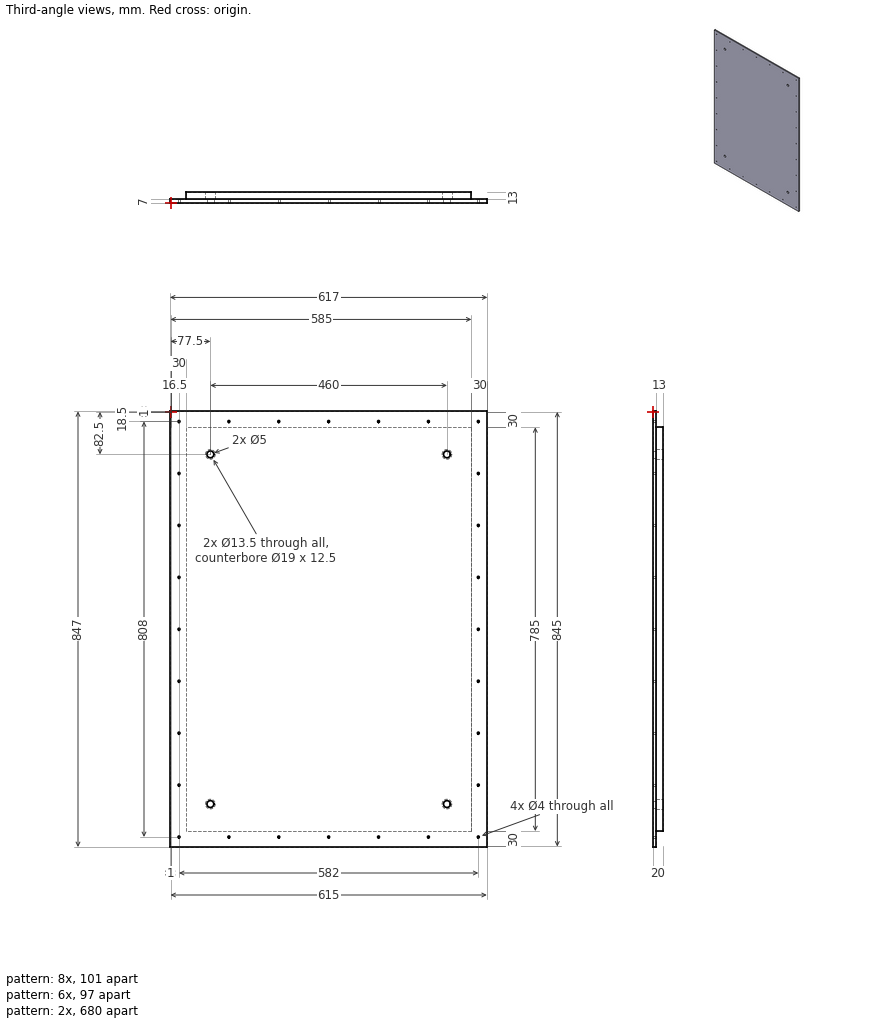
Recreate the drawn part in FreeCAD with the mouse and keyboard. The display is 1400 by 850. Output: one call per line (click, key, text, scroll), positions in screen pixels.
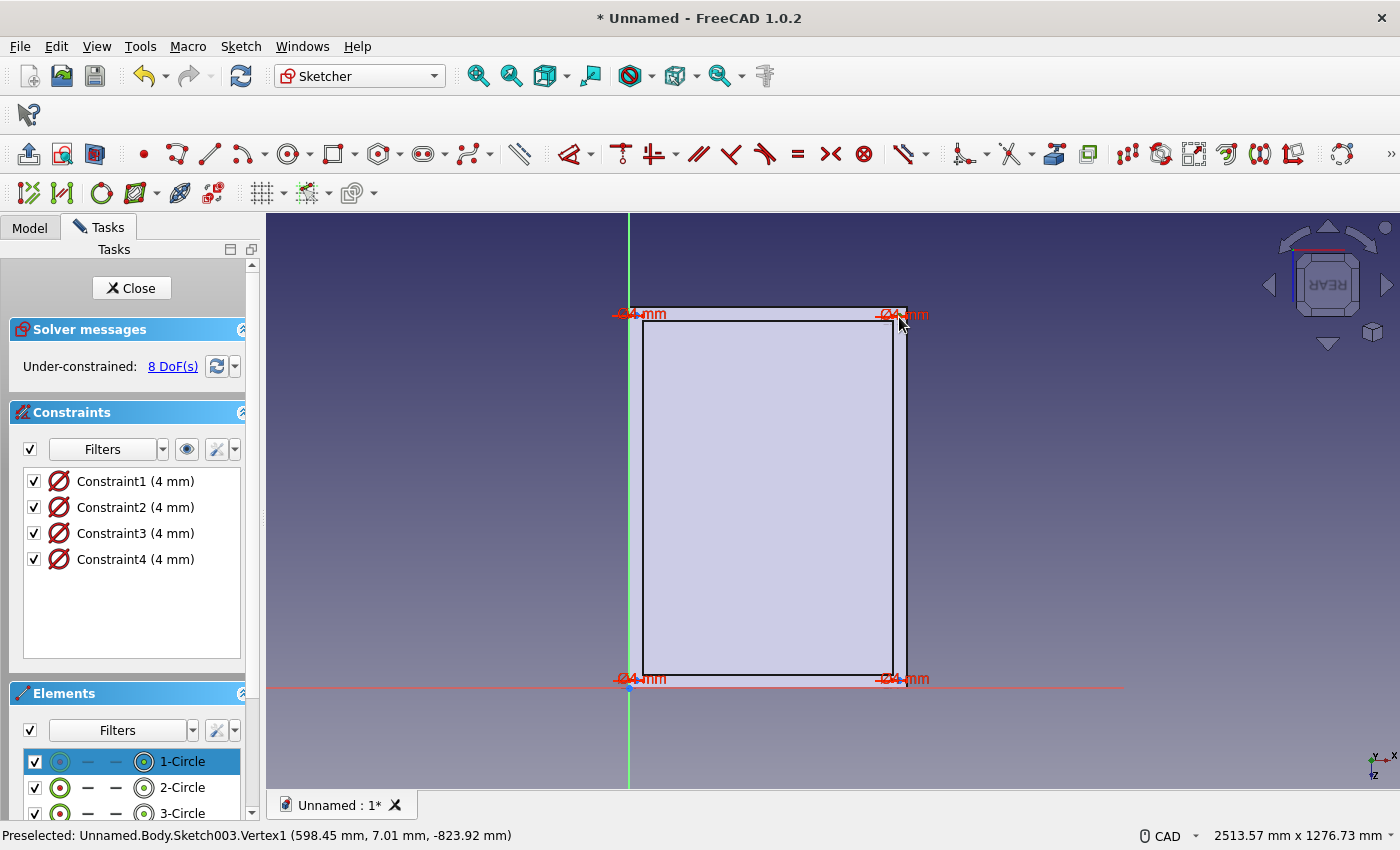
click(637, 316)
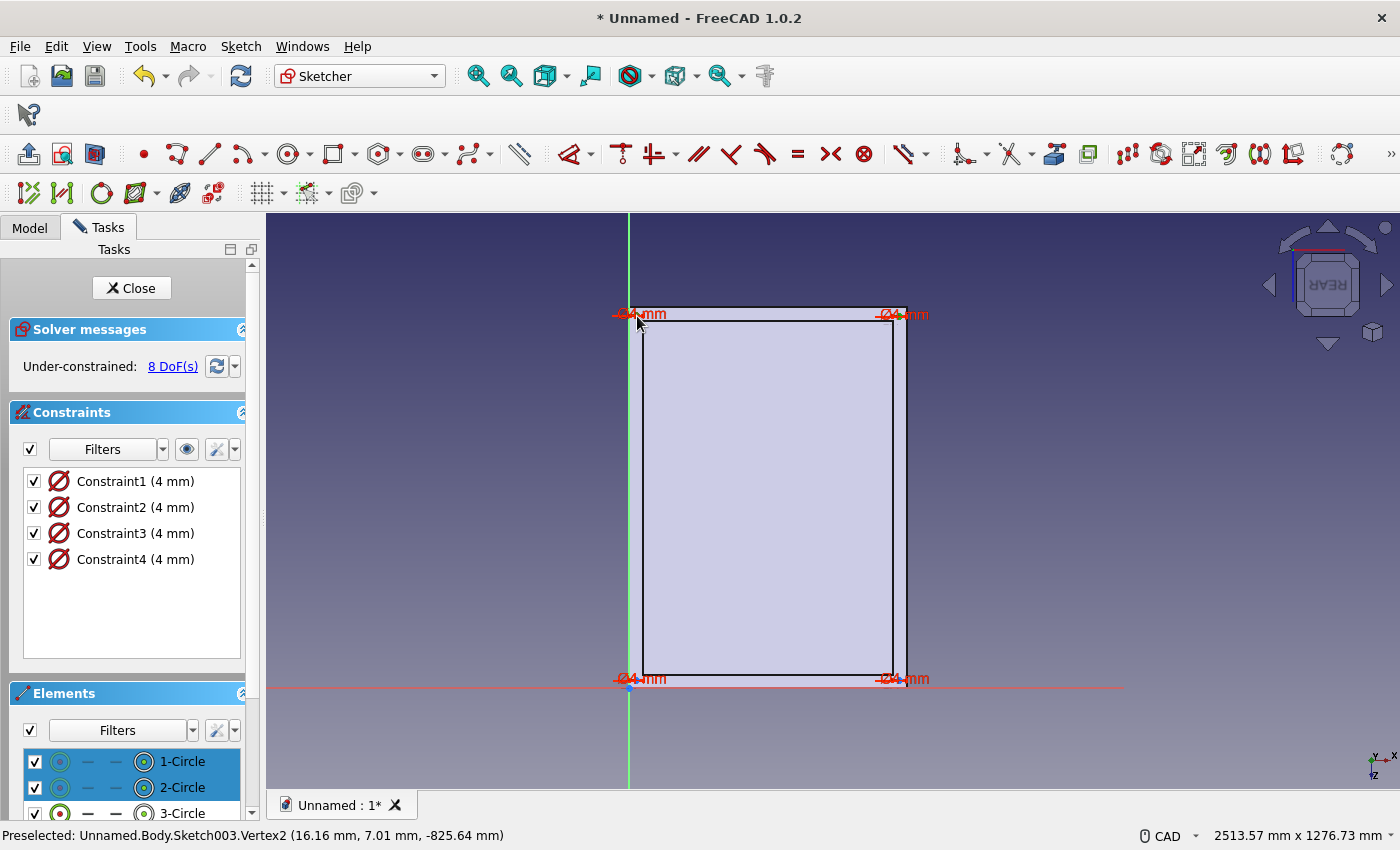
key(h)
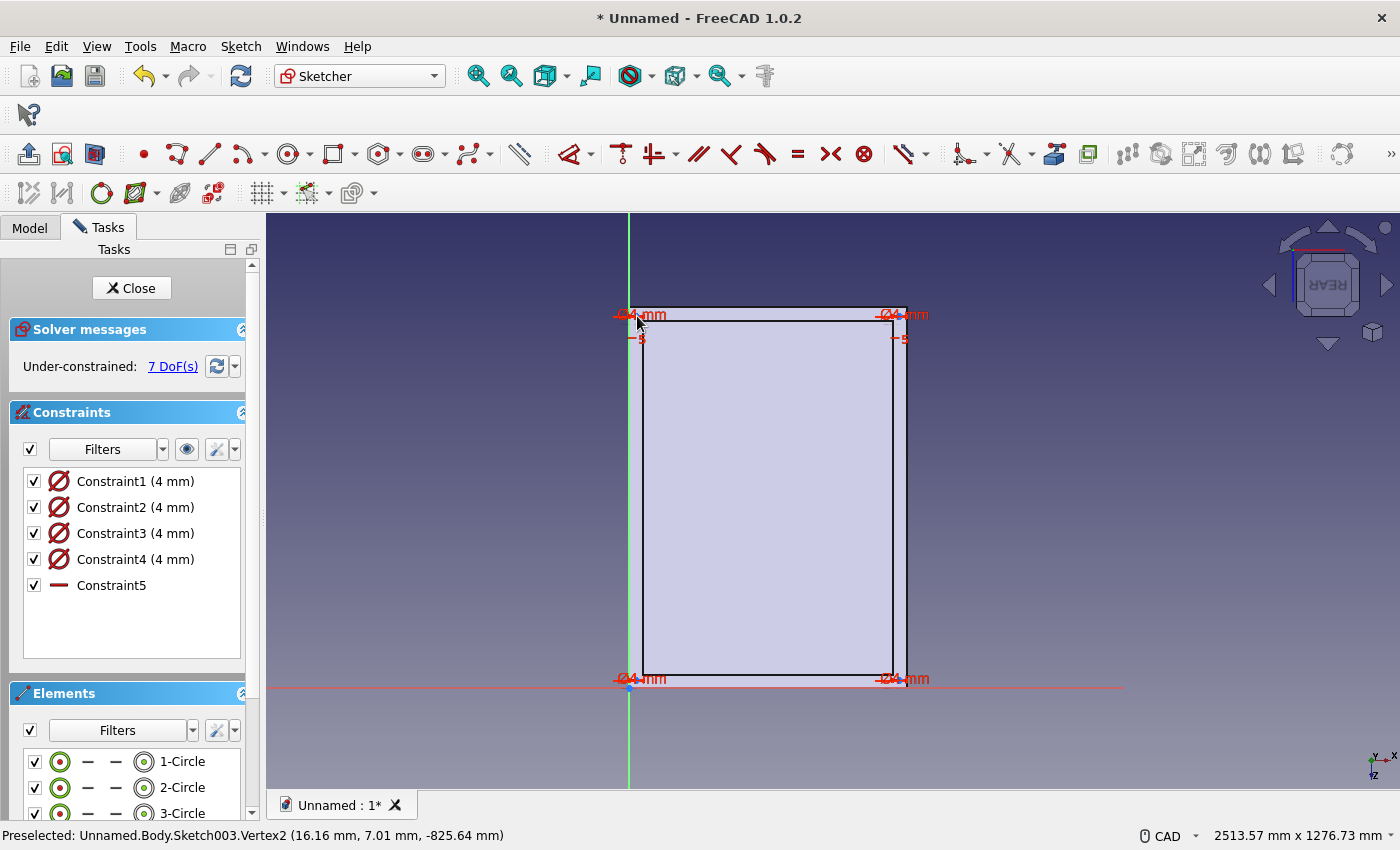
click(637, 317)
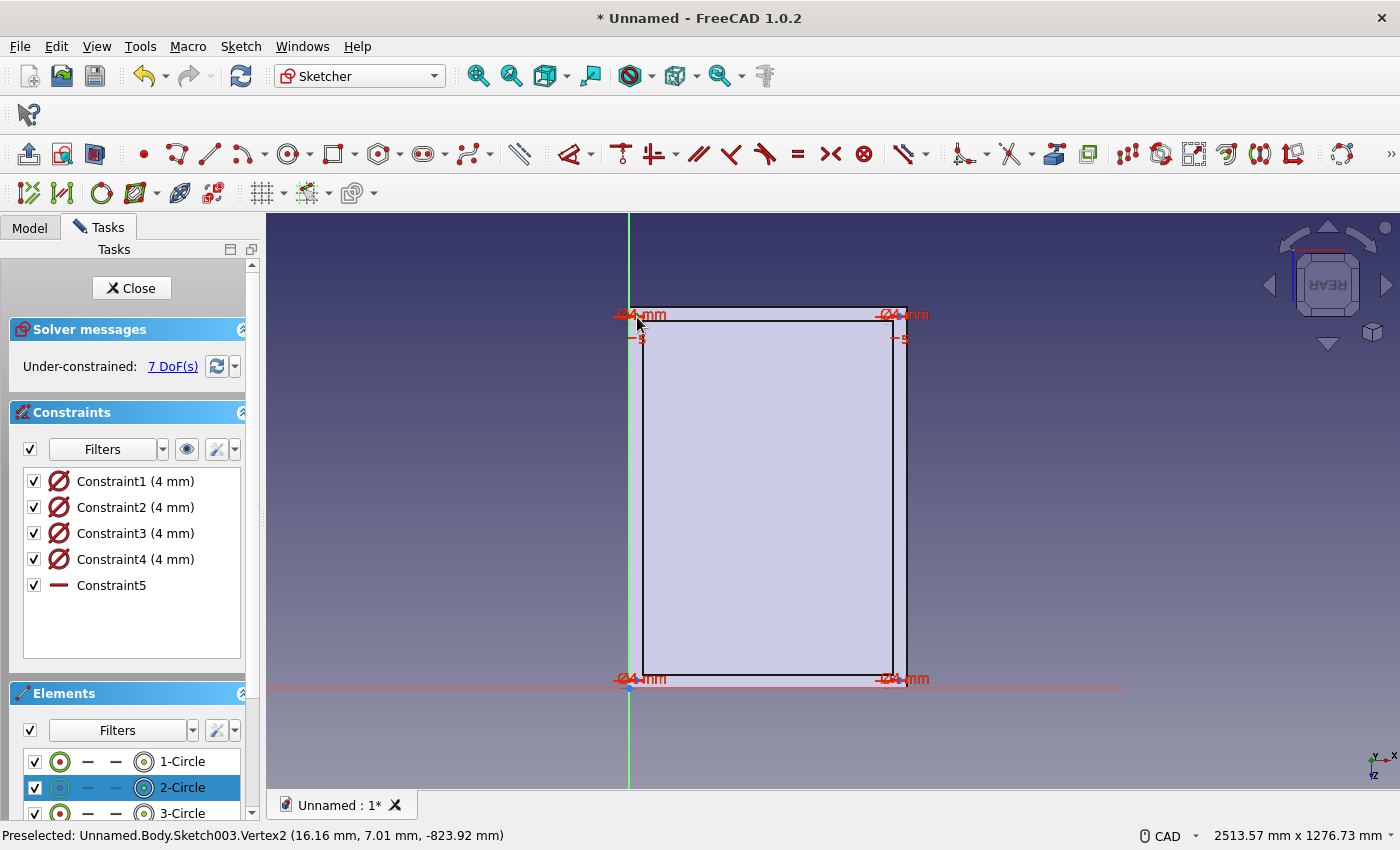
click(637, 681)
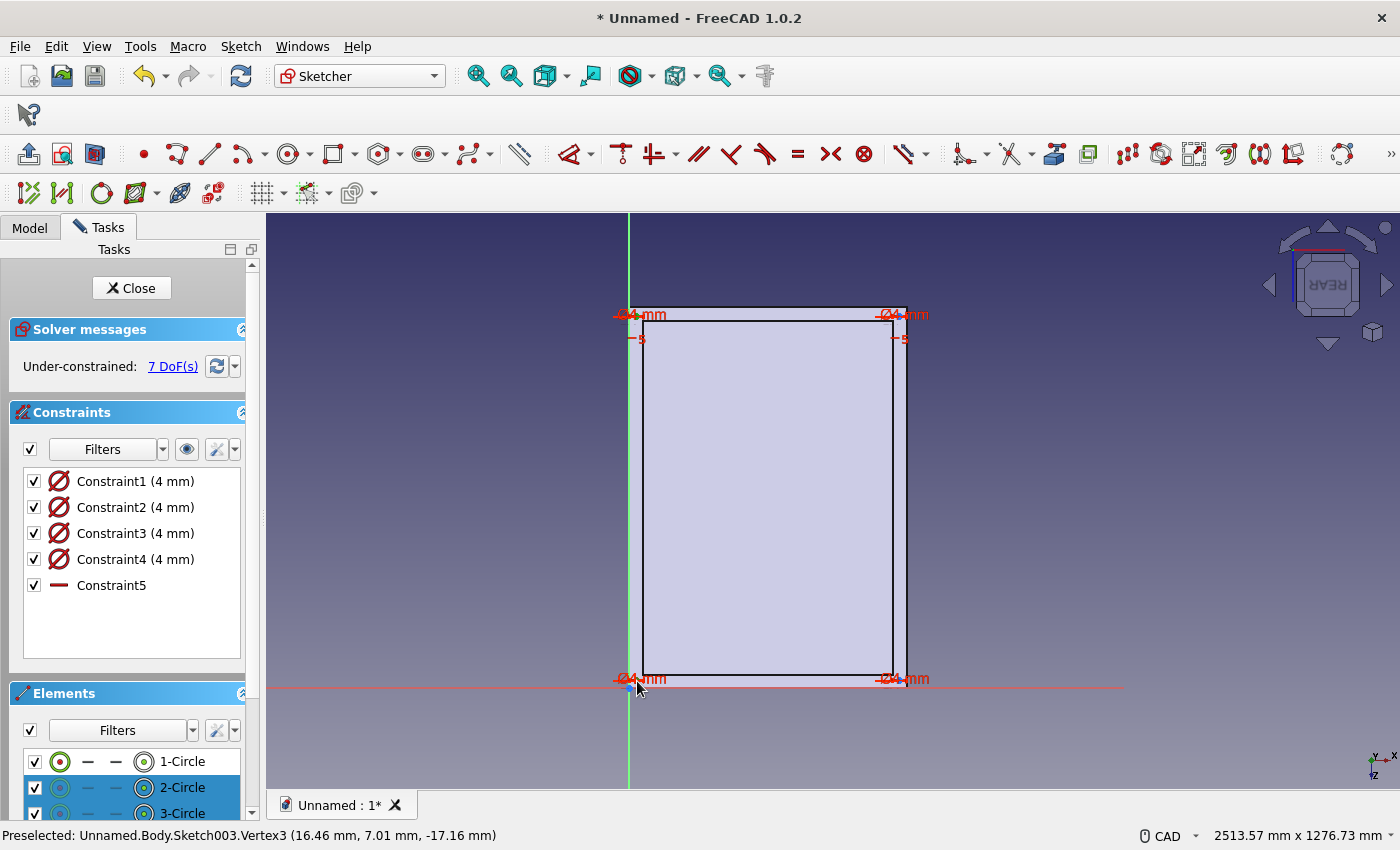
key(v)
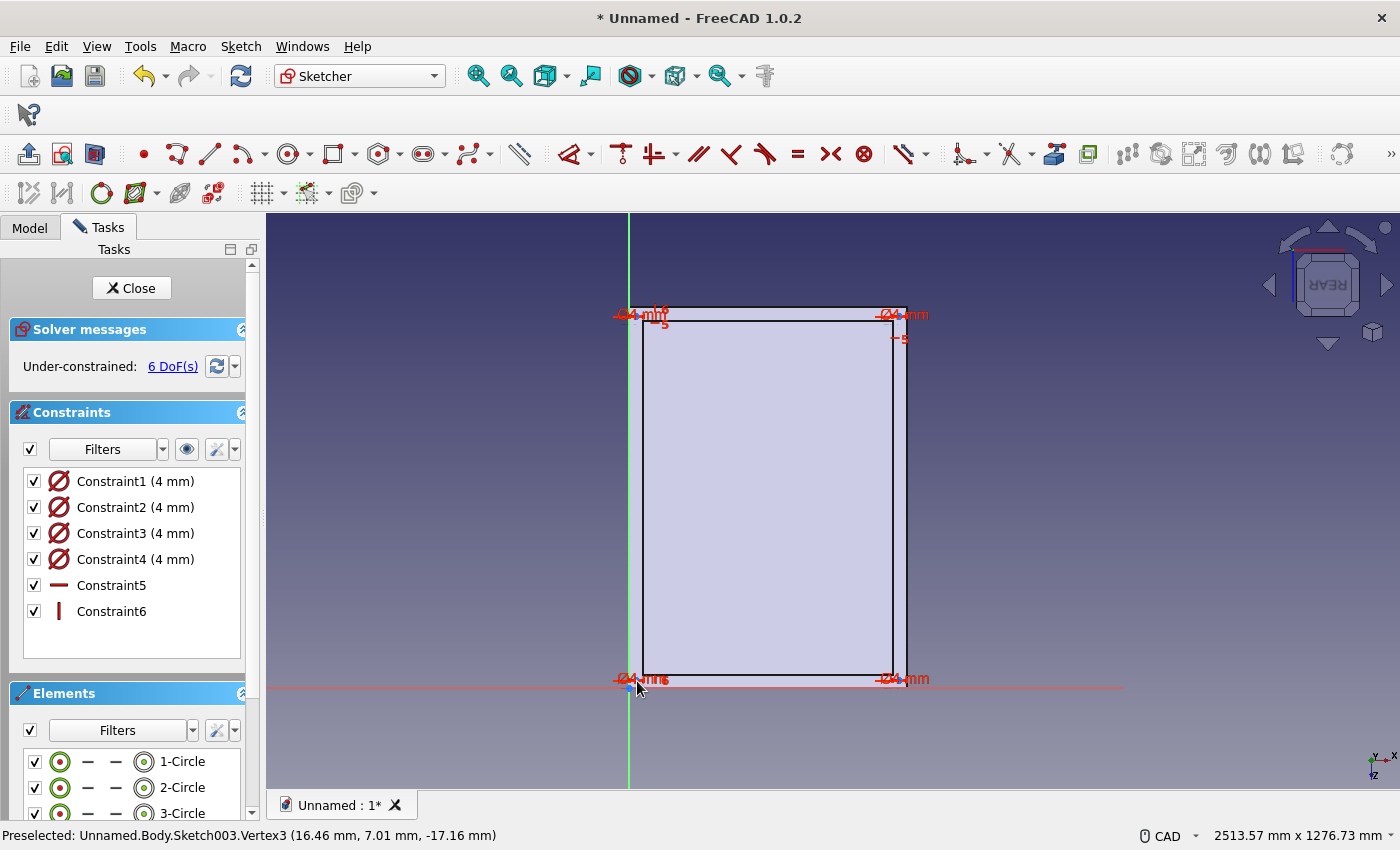
click(899, 317)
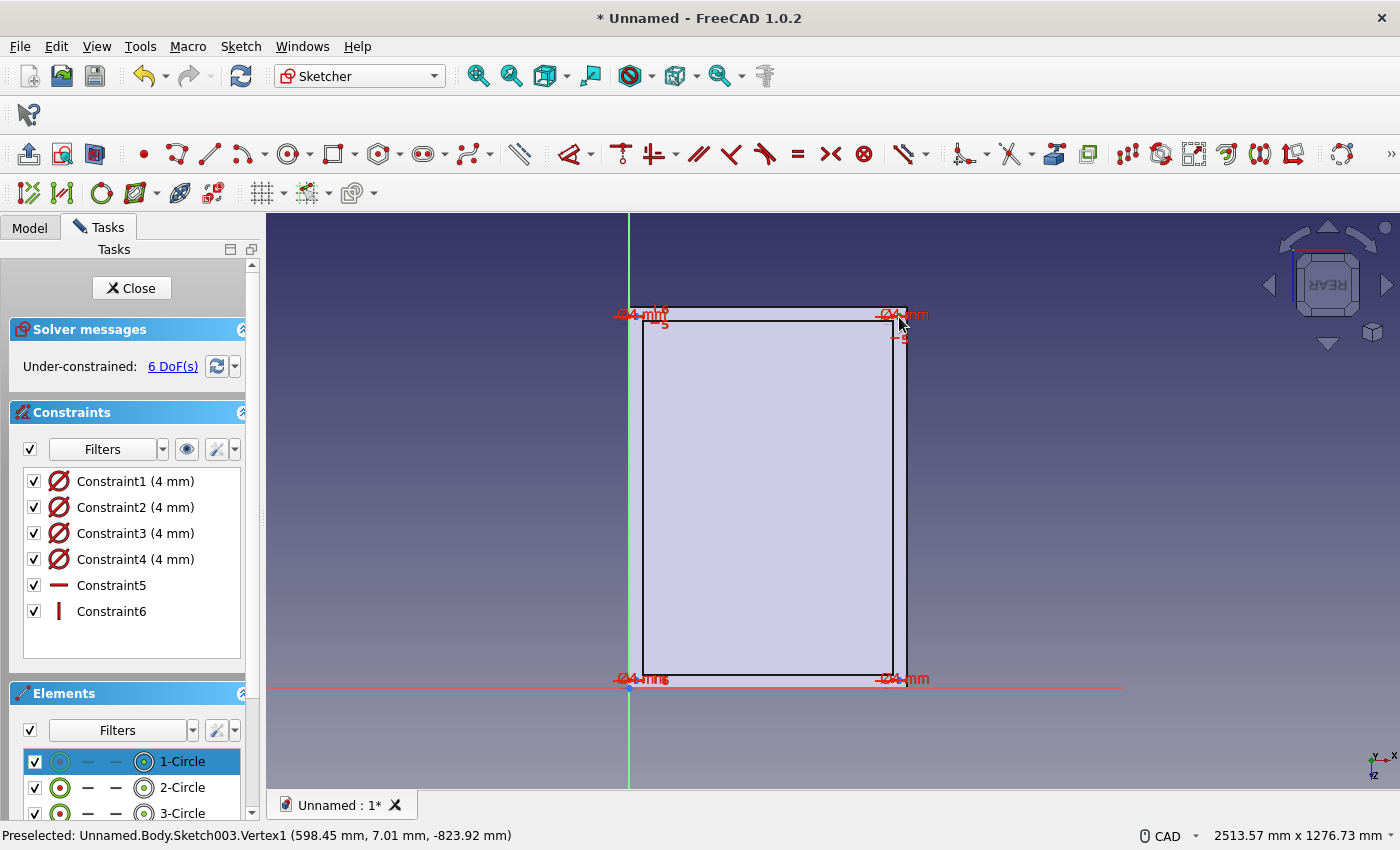
click(900, 681)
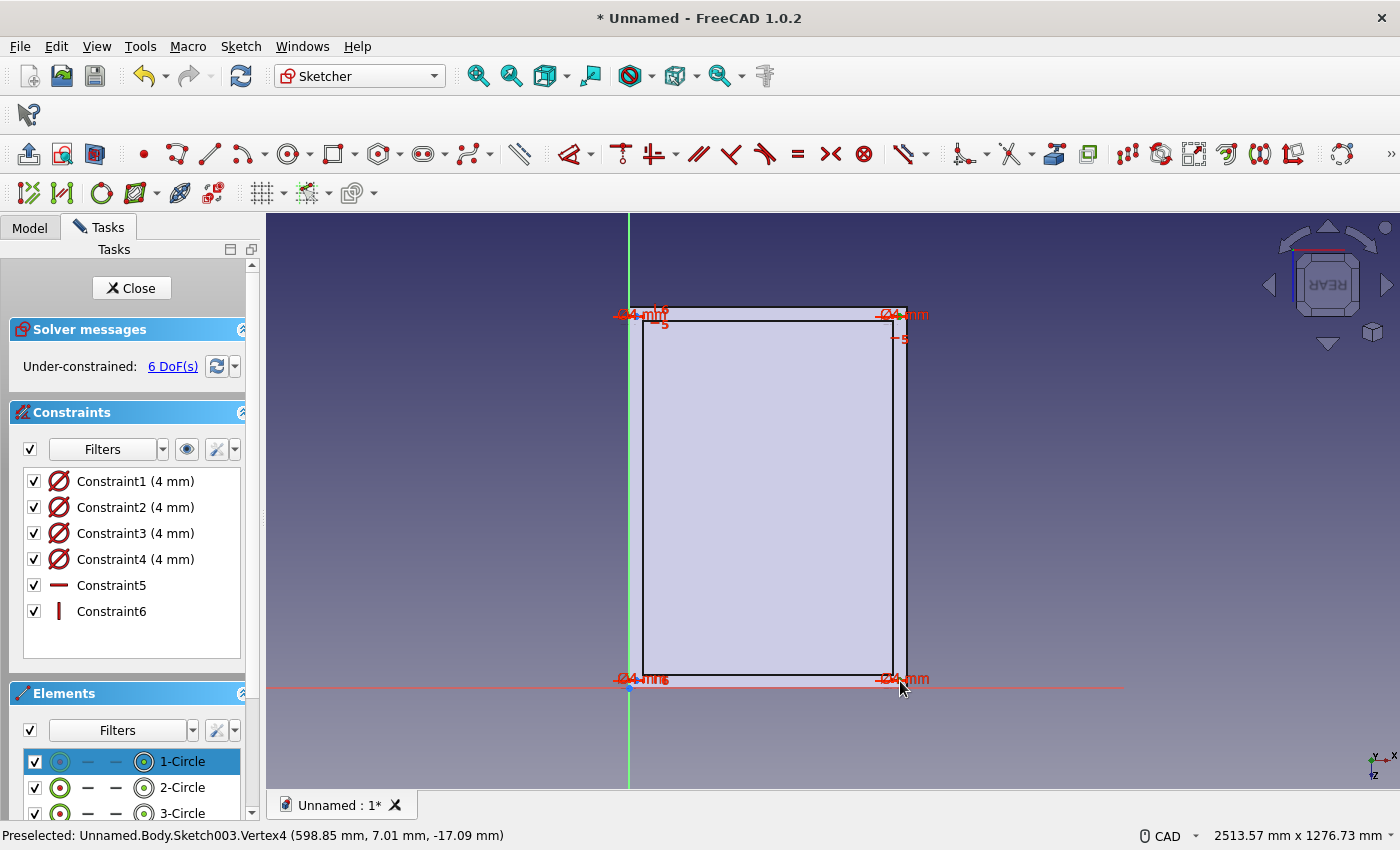
key(v)